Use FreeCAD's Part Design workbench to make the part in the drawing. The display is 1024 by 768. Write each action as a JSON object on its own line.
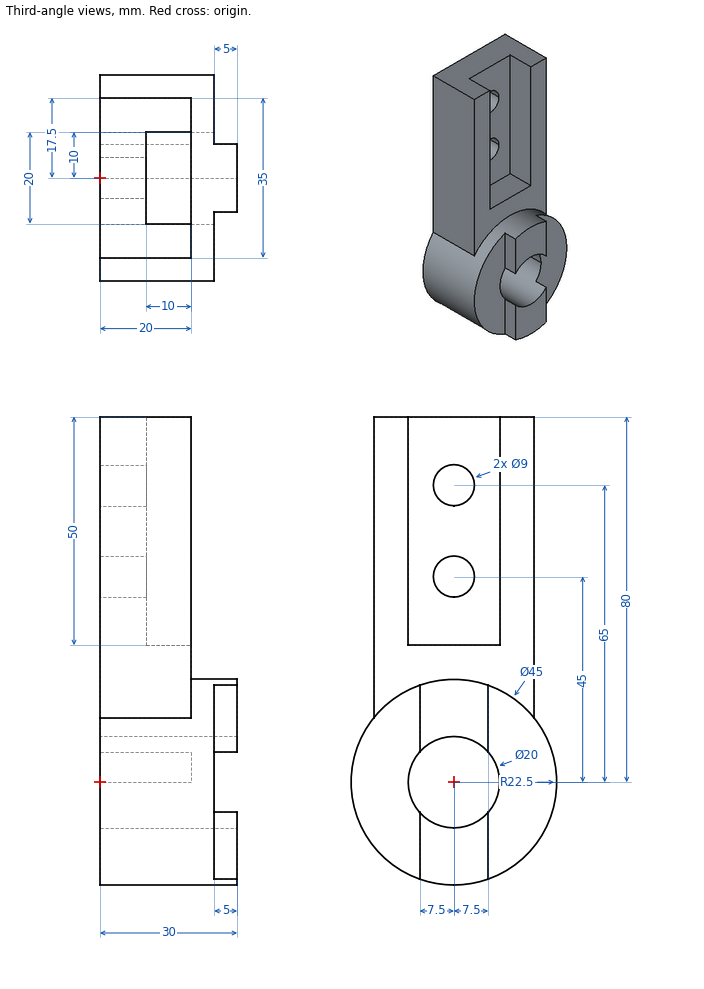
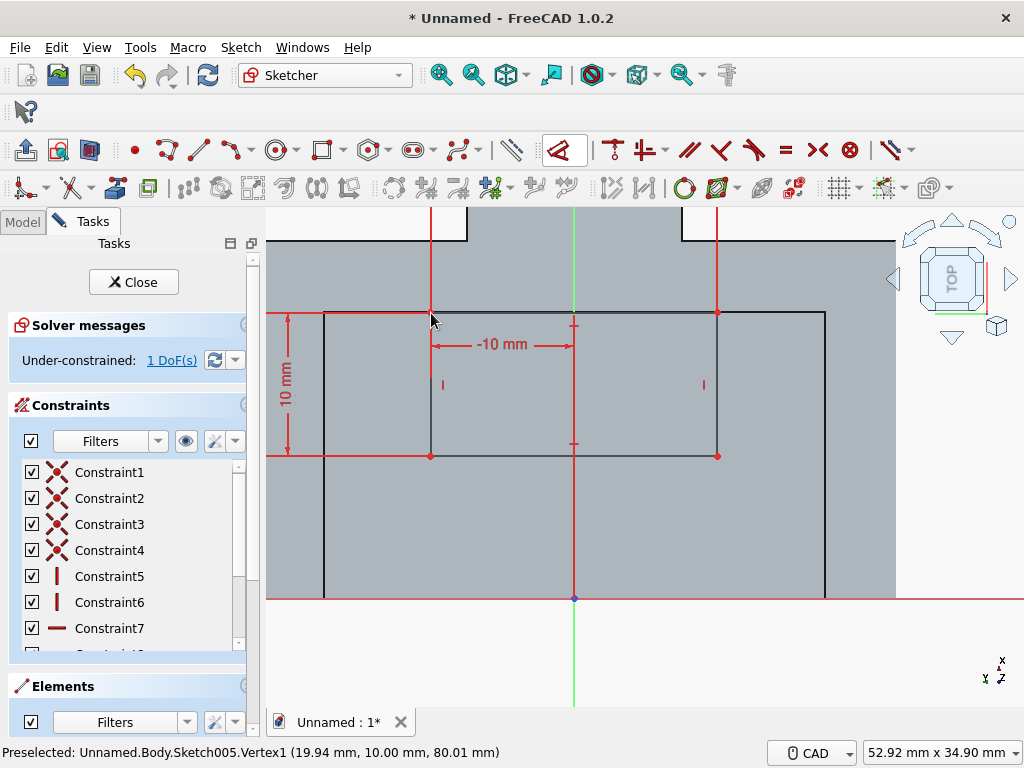
{"action": "left_click", "coordinate": [431, 313]}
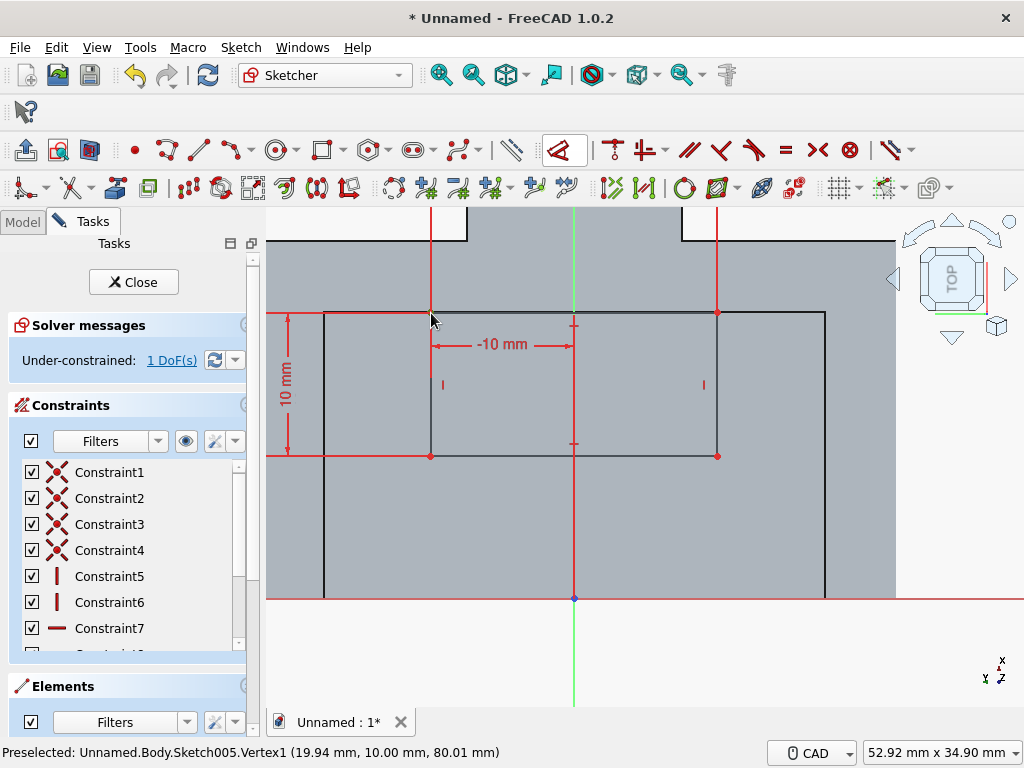
{"action": "left_click", "coordinate": [582, 150]}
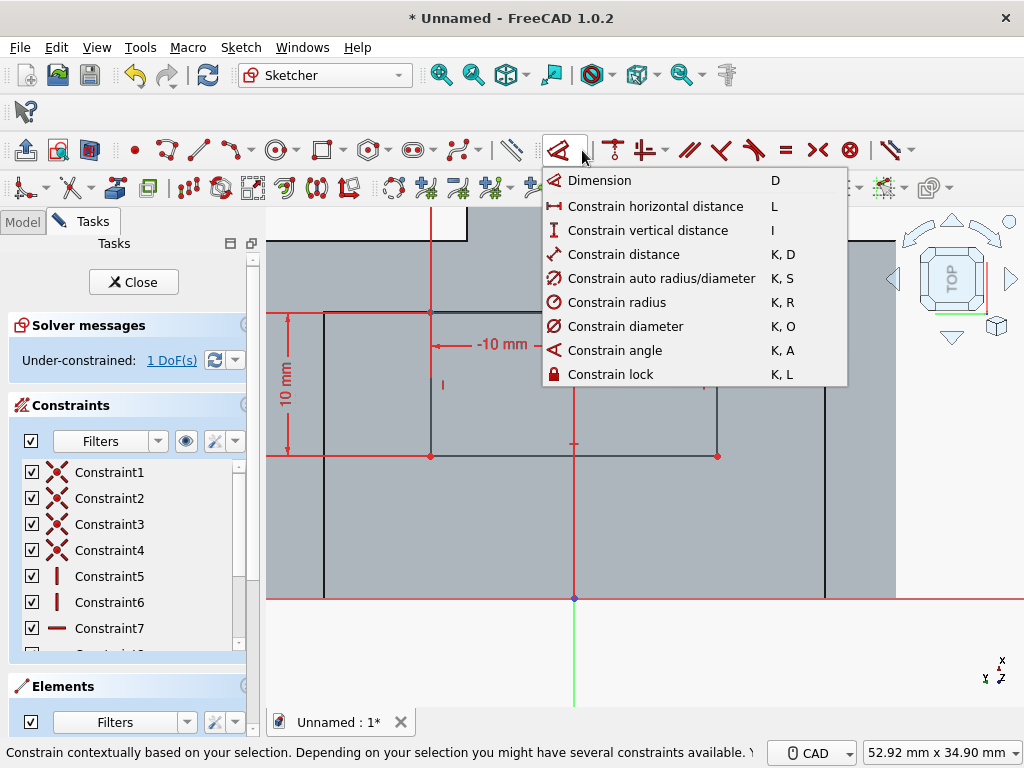
{"action": "left_click", "coordinate": [695, 230]}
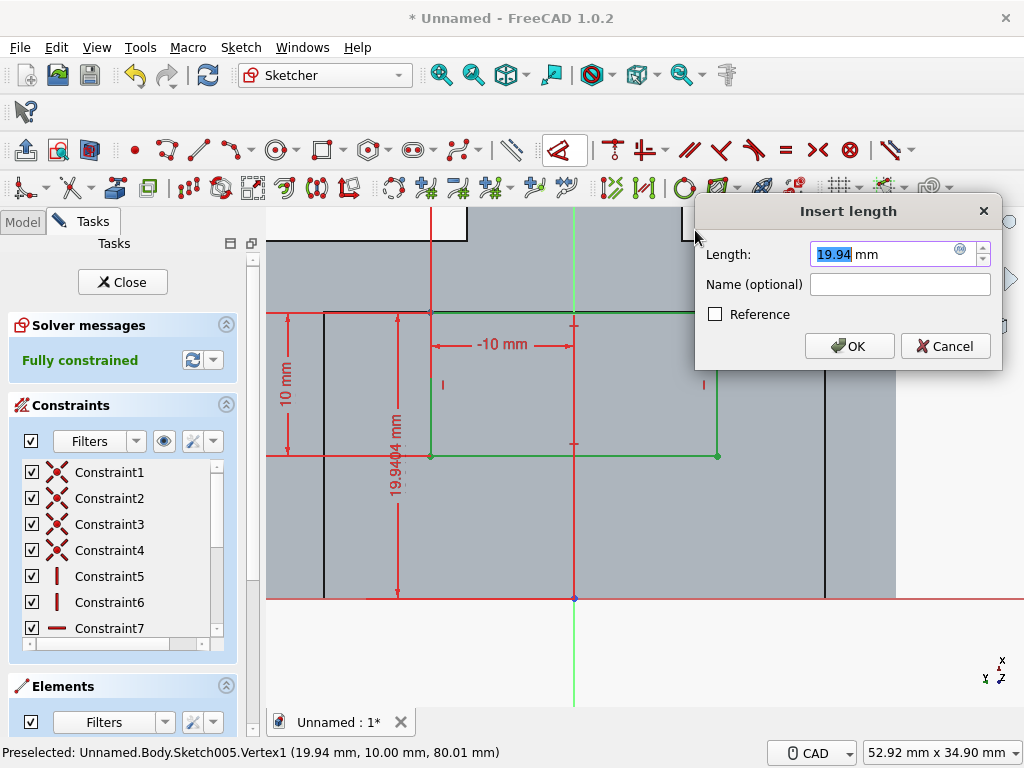
{"action": "type", "text": "20"}
{"action": "key", "text": "Return"}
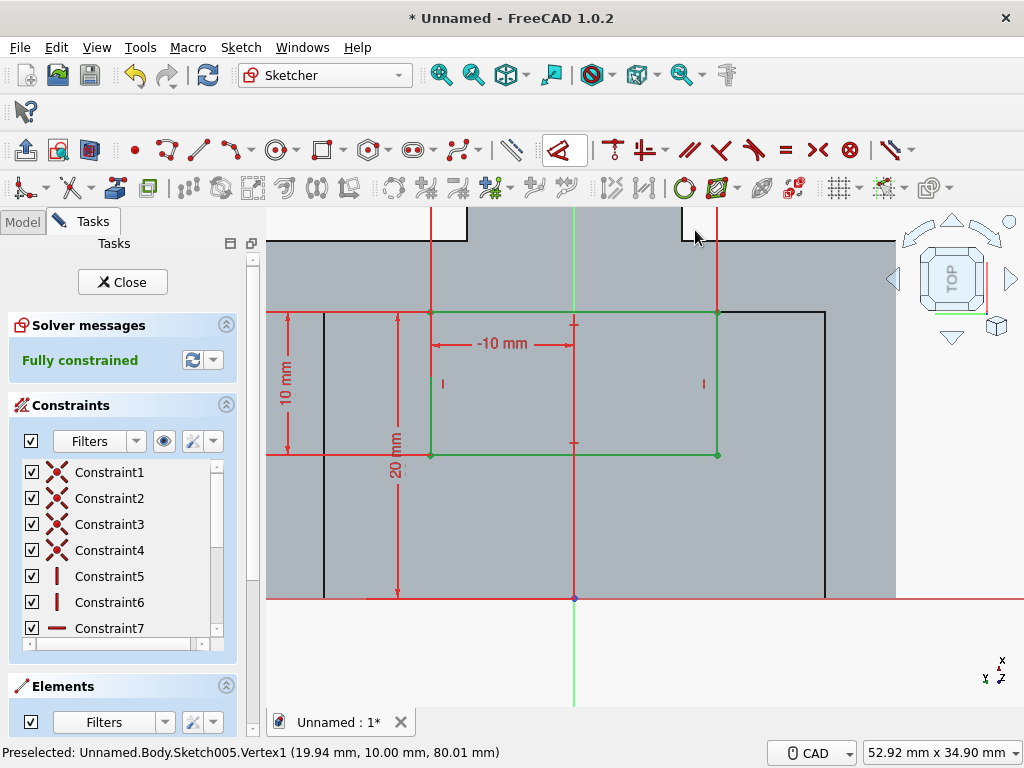
{"action": "left_click", "coordinate": [123, 282]}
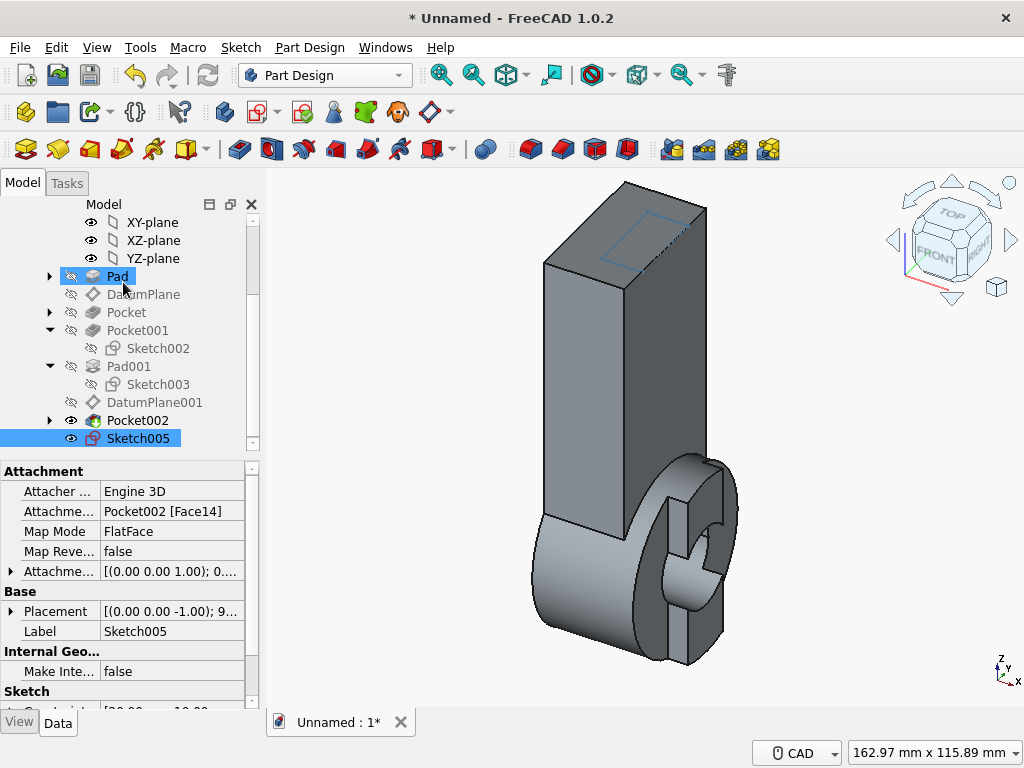
{"action": "left_click", "coordinate": [240, 150]}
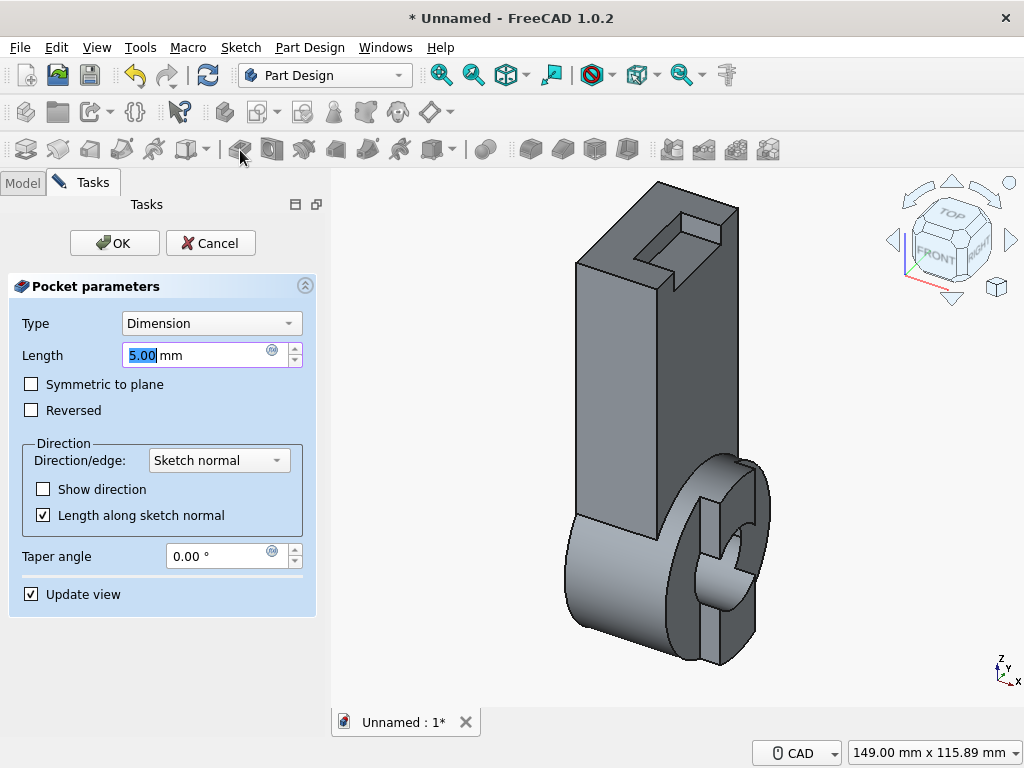
{"action": "type", "text": "50"}
{"action": "key", "text": "Tab"}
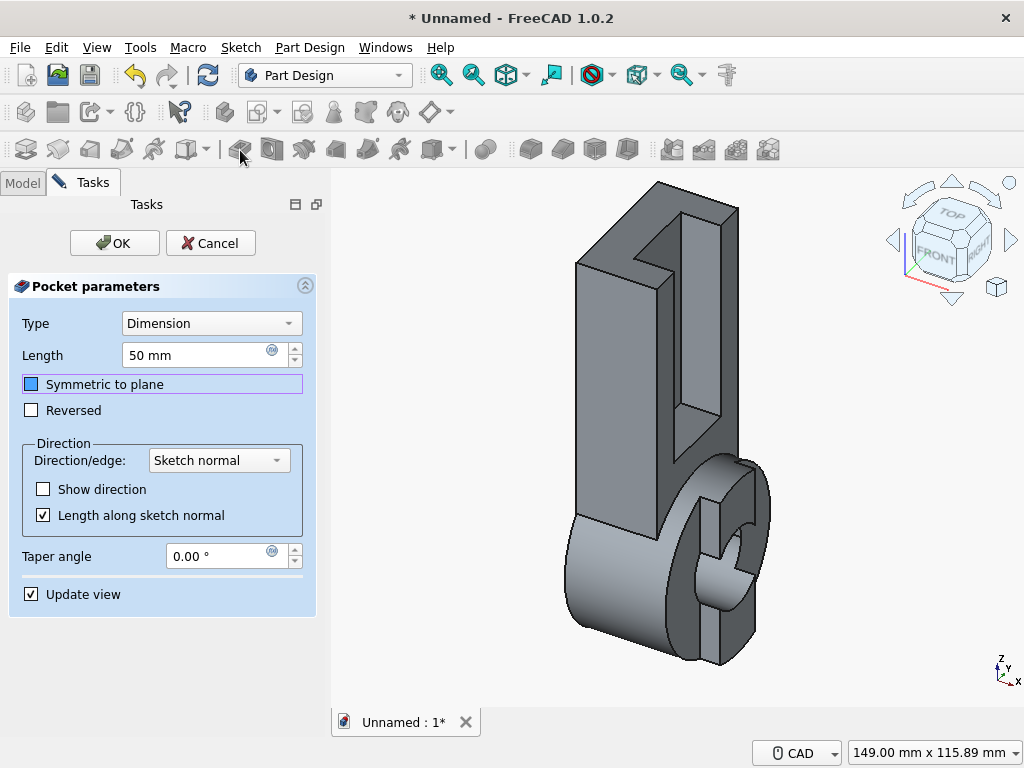
{"action": "left_click", "coordinate": [115, 243]}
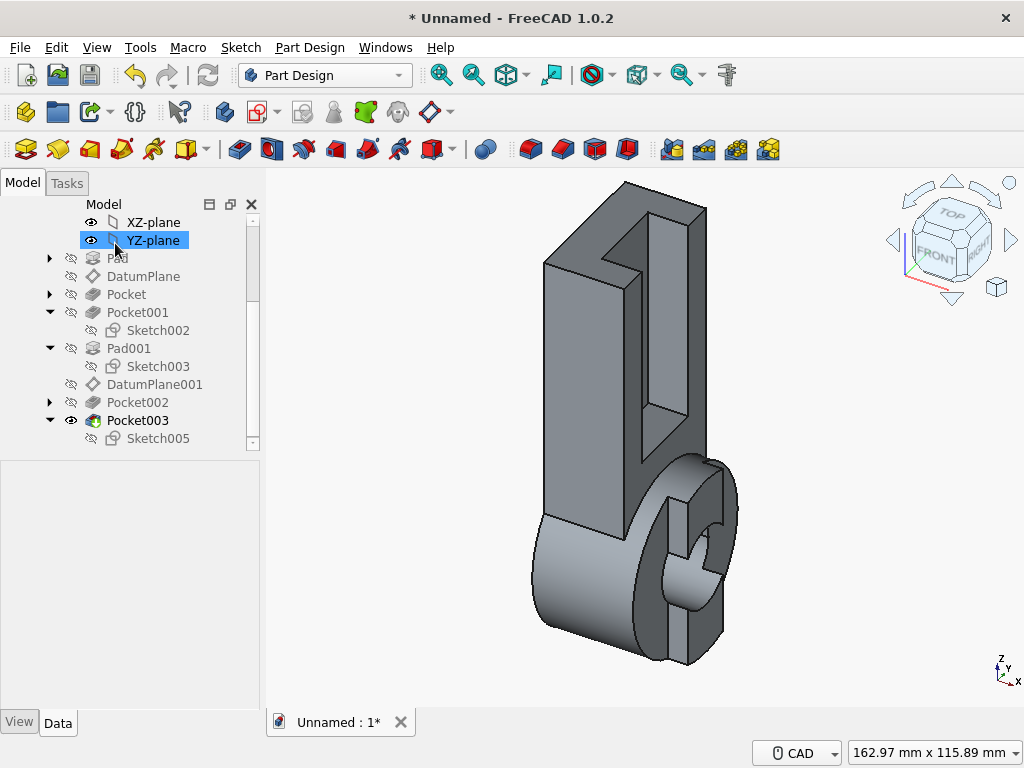
{"action": "key", "text": "0"}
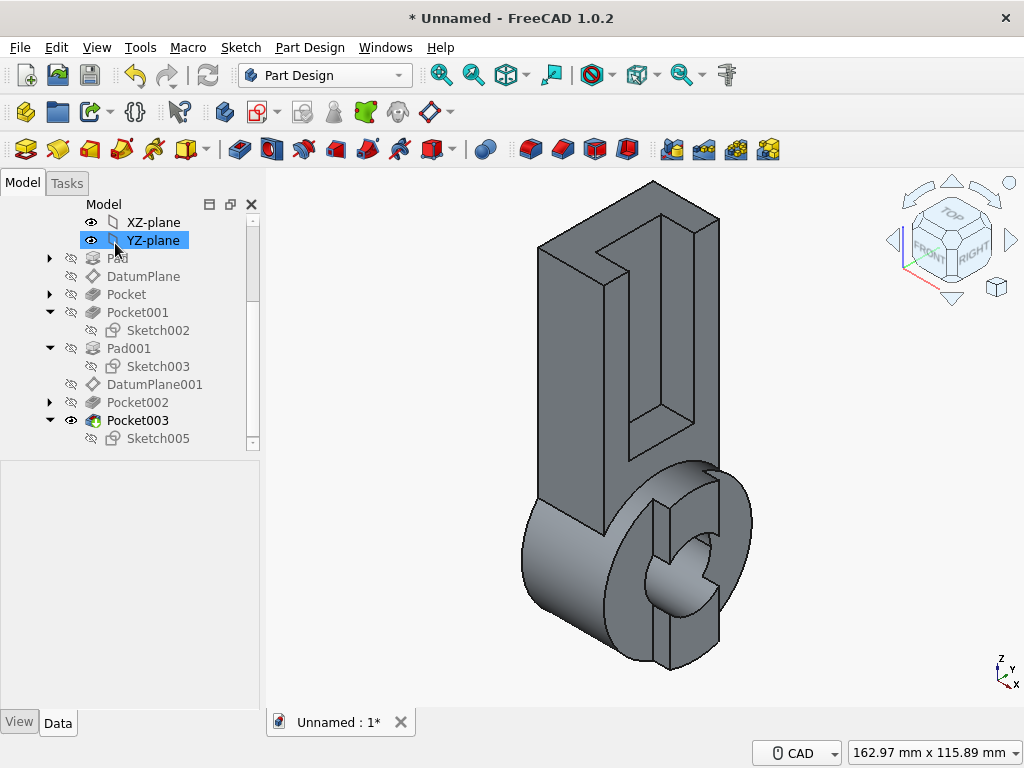
{"action": "left_click", "coordinate": [638, 376]}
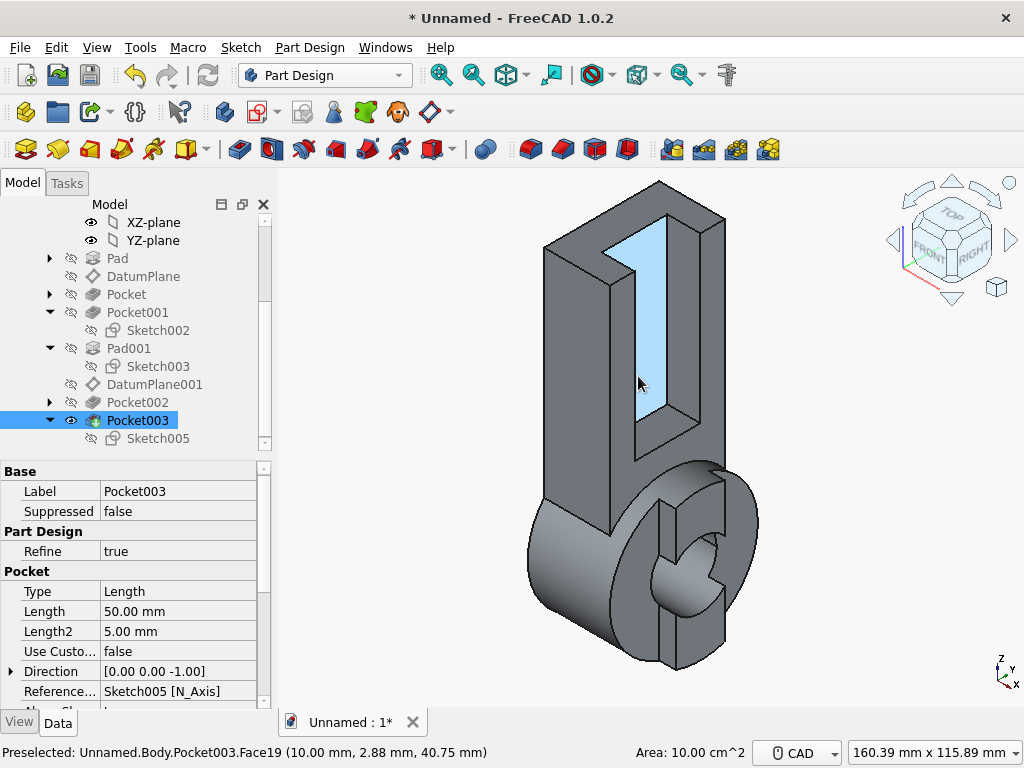
{"action": "left_click", "coordinate": [258, 112]}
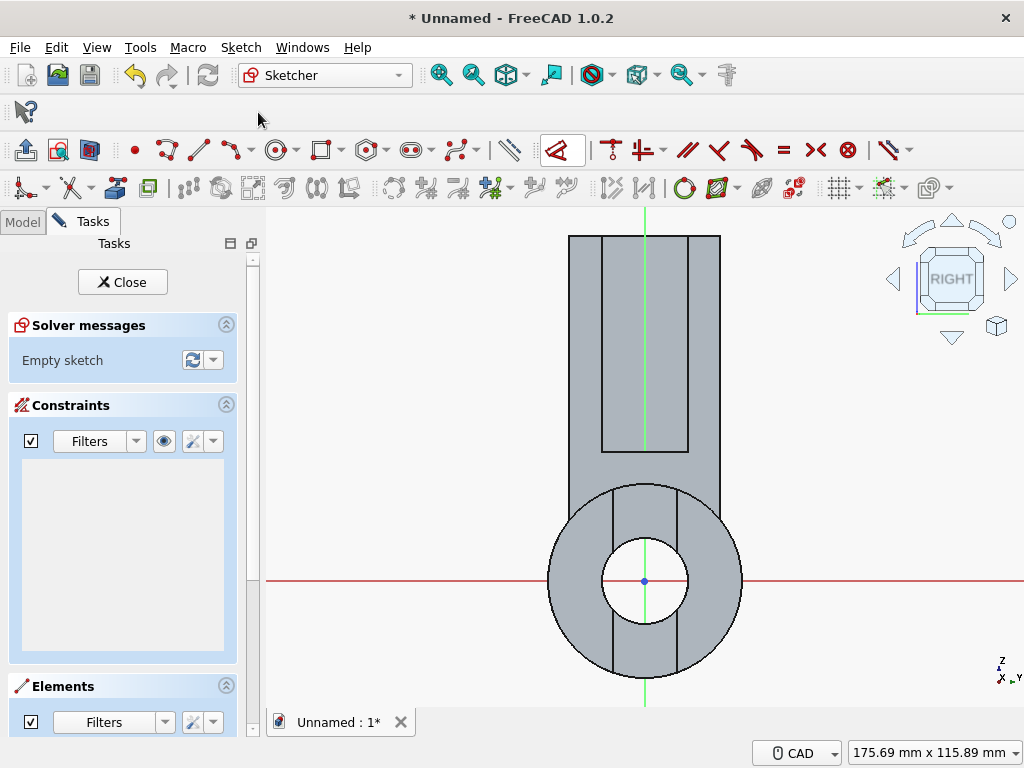
{"action": "left_click", "coordinate": [90, 150]}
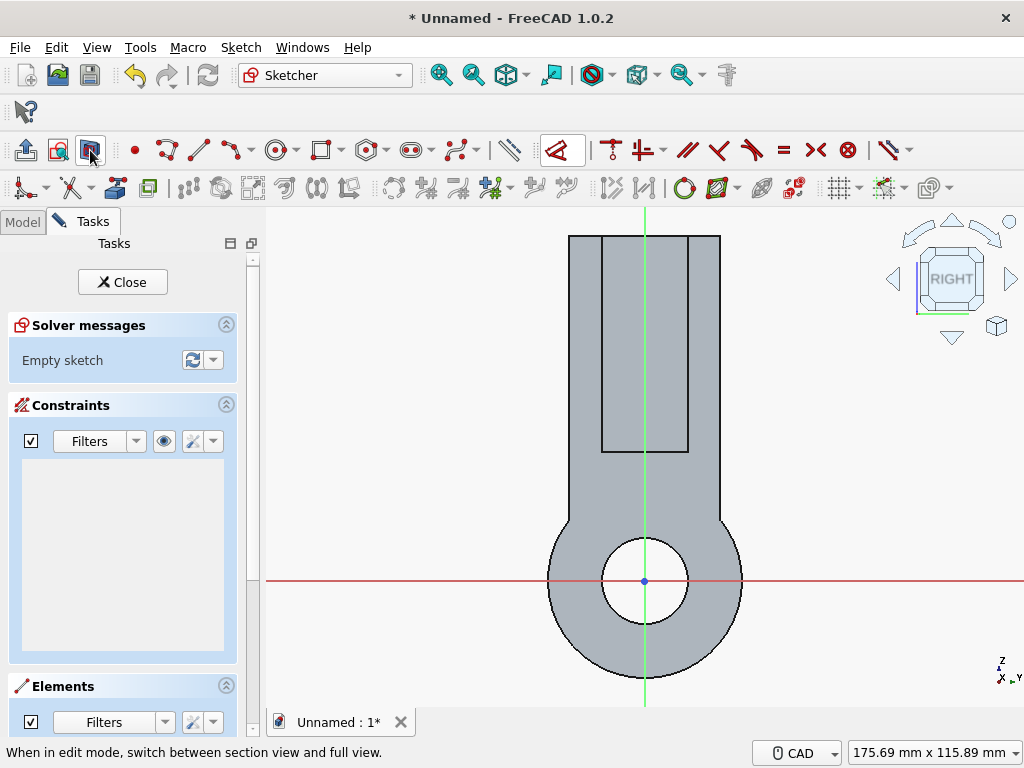
{"action": "left_click", "coordinate": [276, 150]}